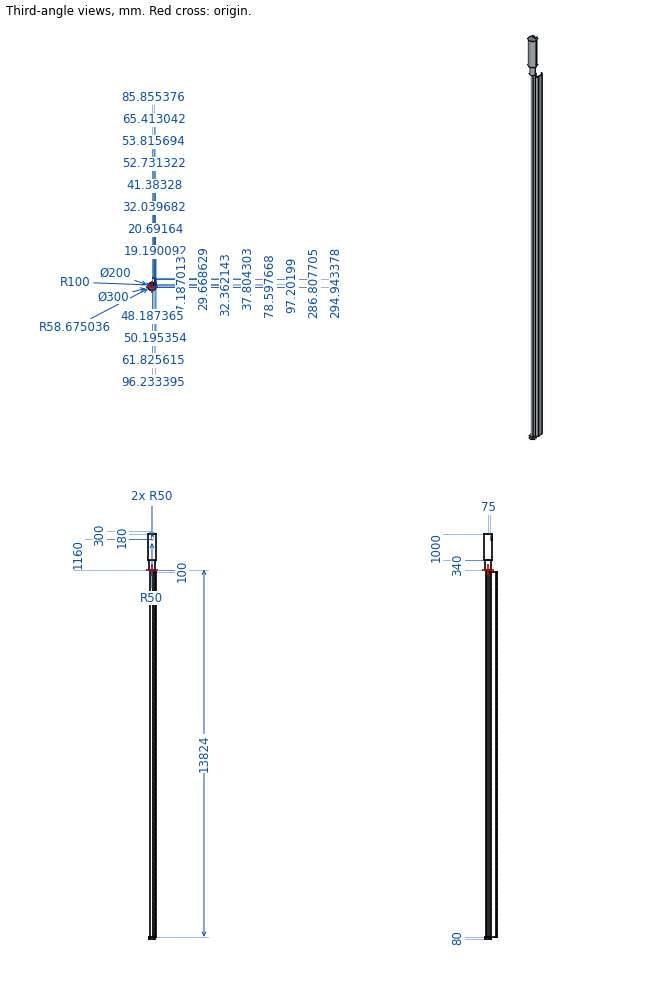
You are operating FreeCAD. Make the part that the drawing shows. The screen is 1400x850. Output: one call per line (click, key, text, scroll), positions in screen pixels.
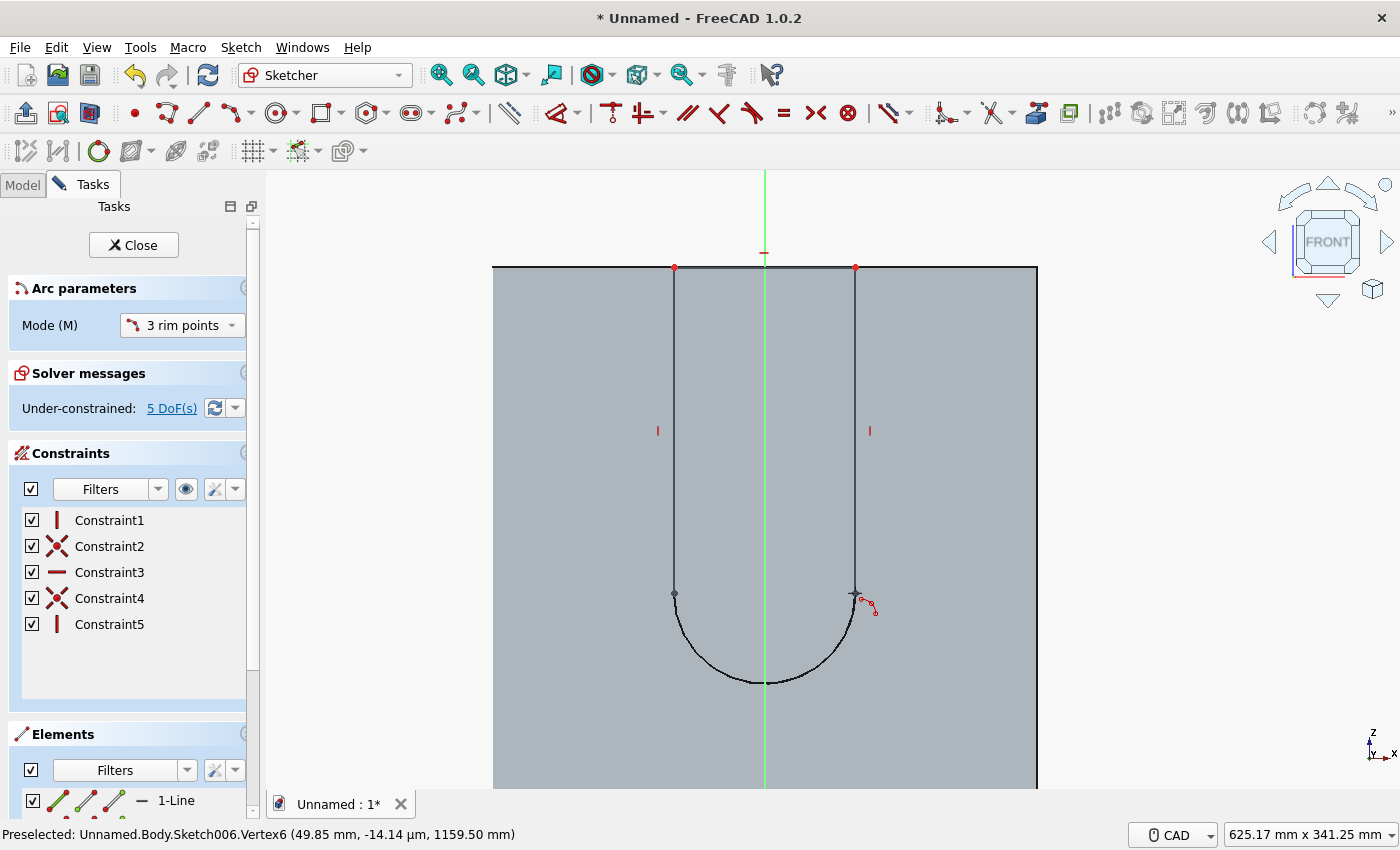
click(855, 594)
click(674, 594)
click(737, 679)
key(Escape)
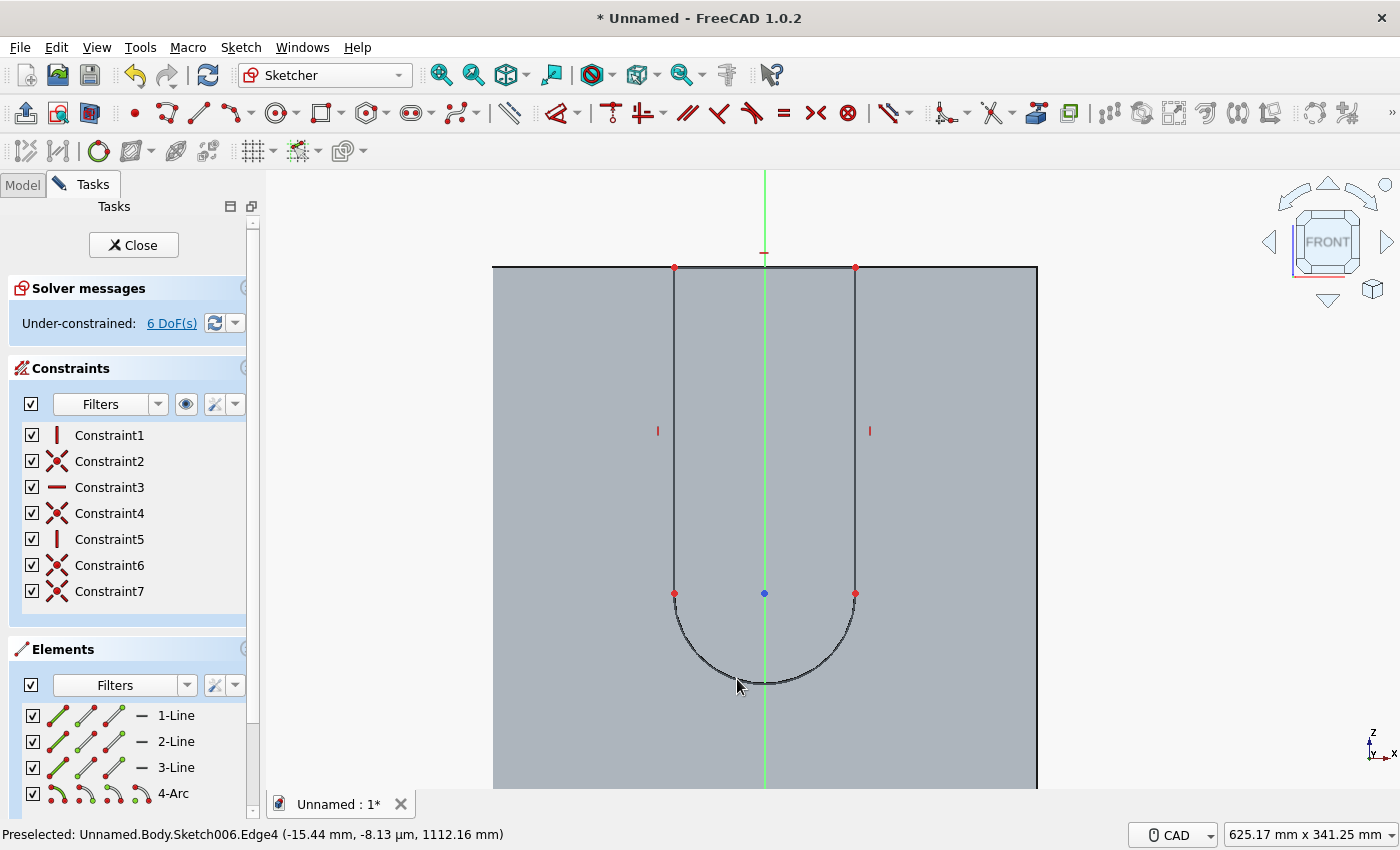
click(764, 594)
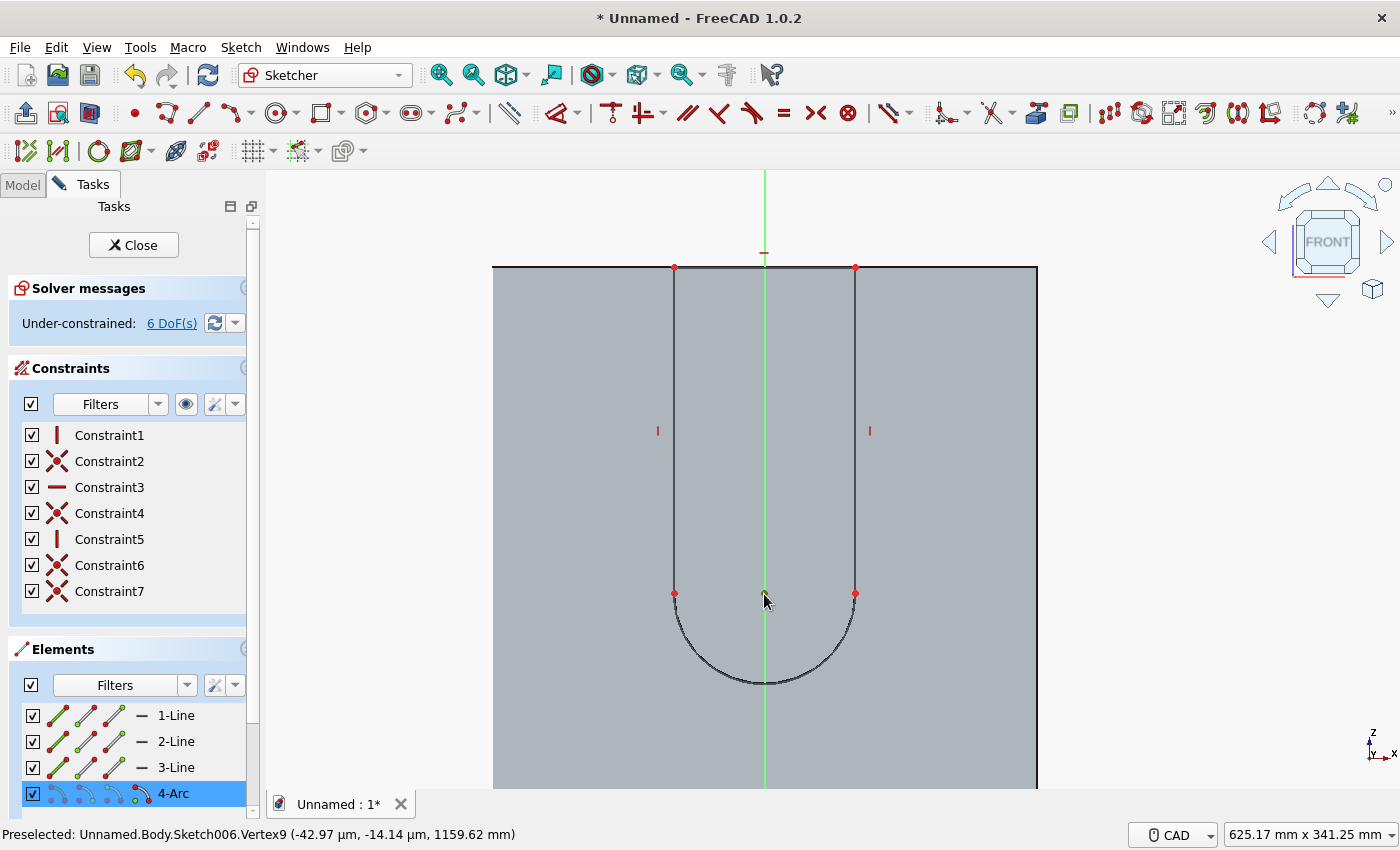
click(765, 721)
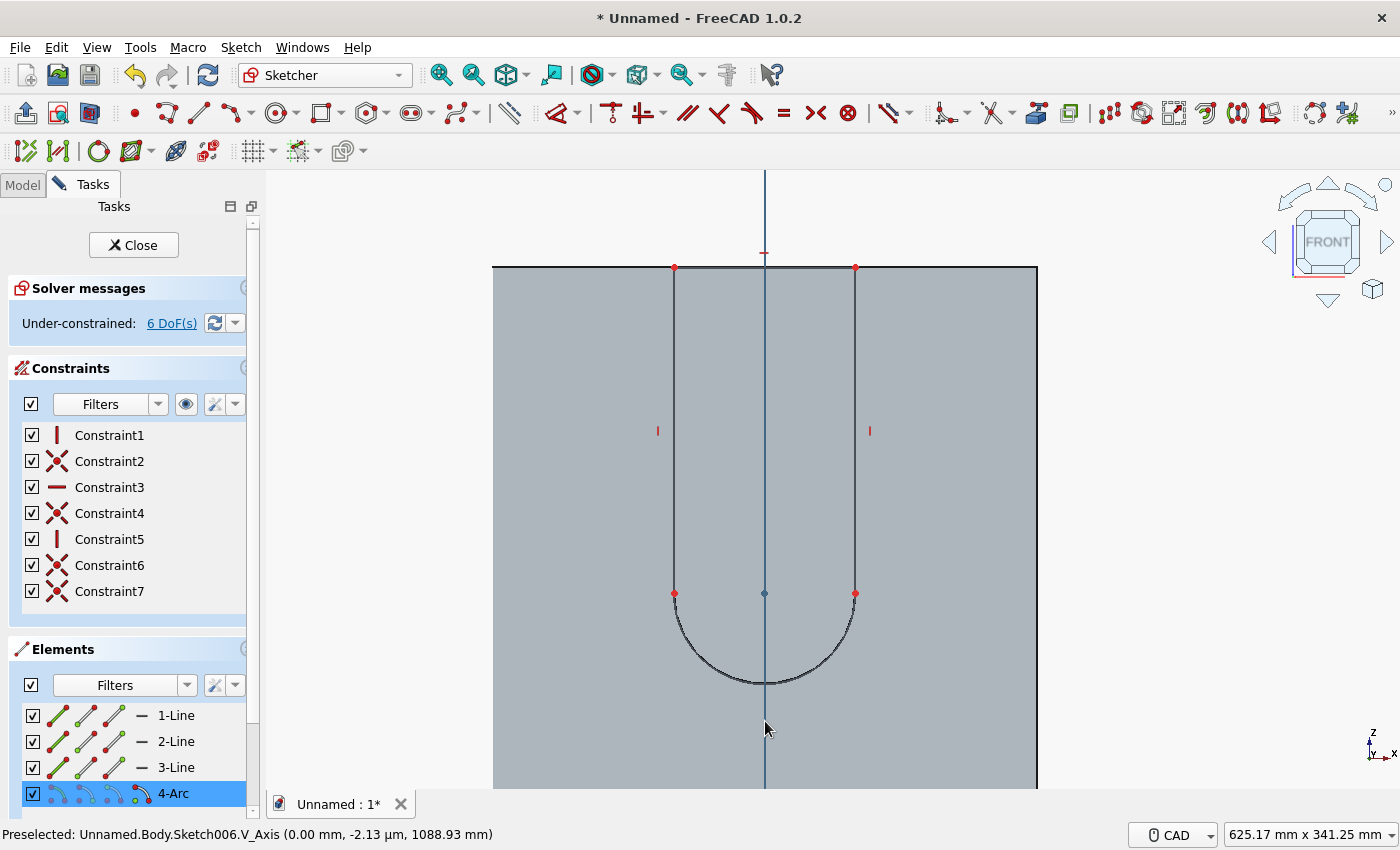
key(c)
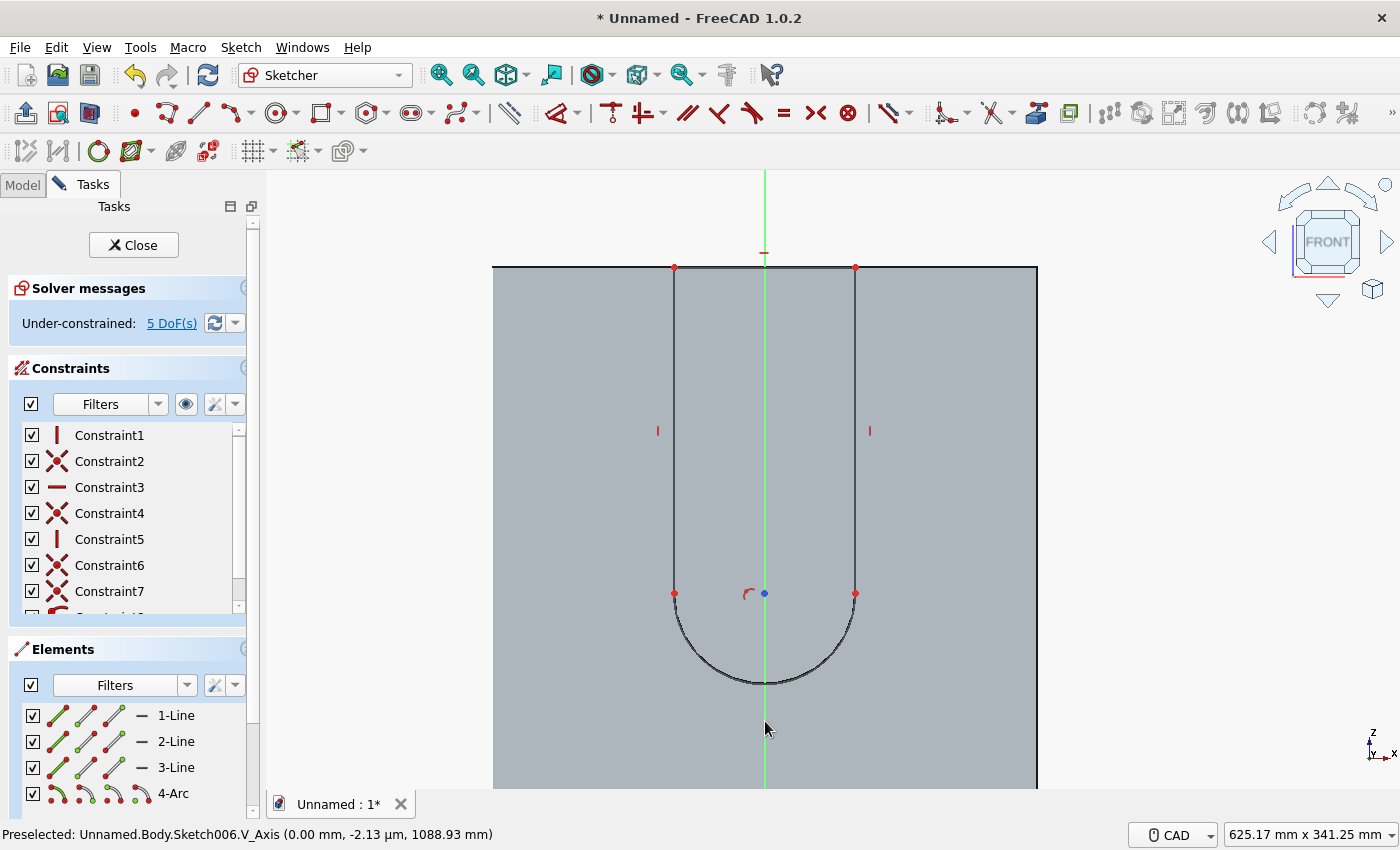
key(d)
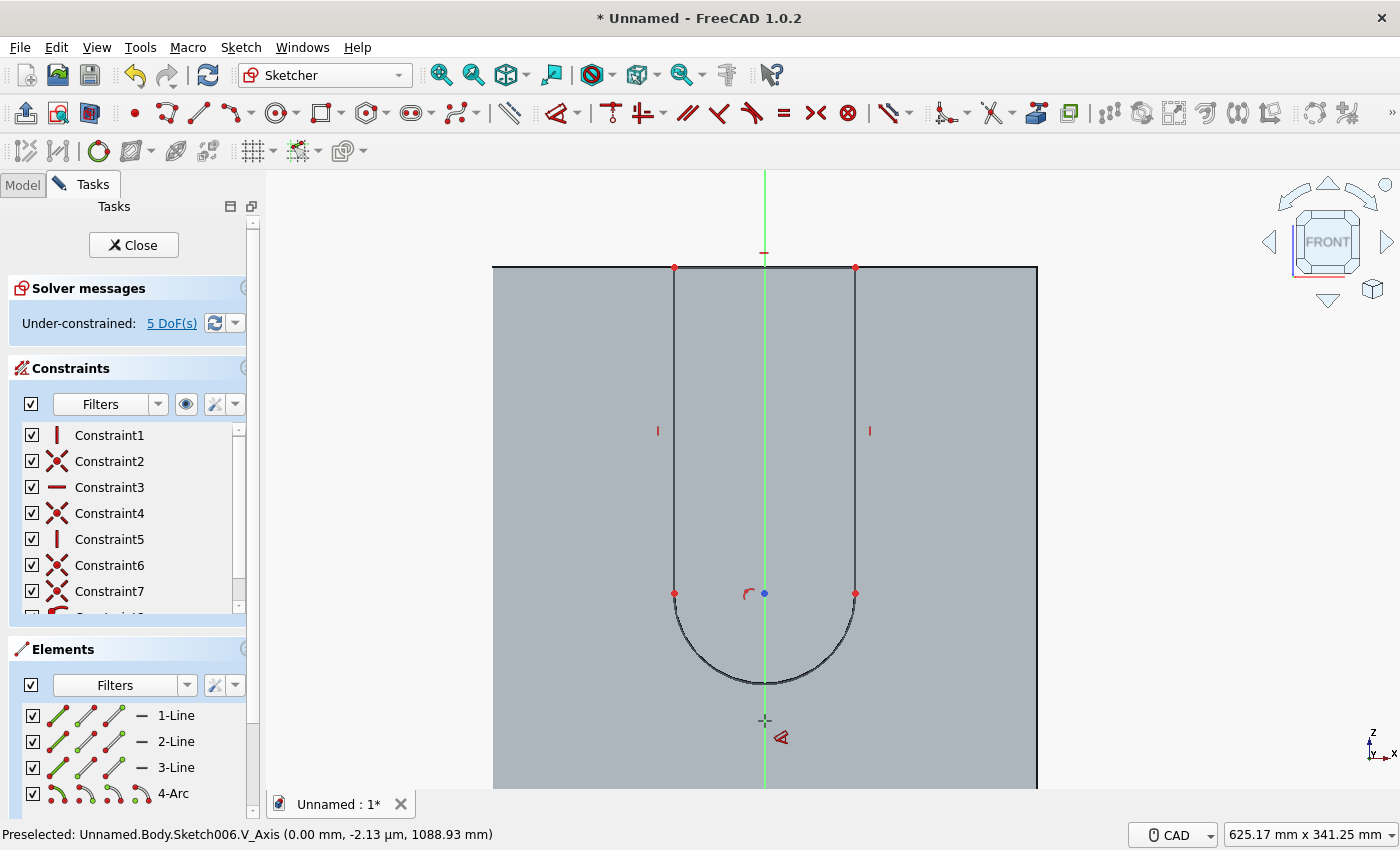
click(711, 667)
click(692, 693)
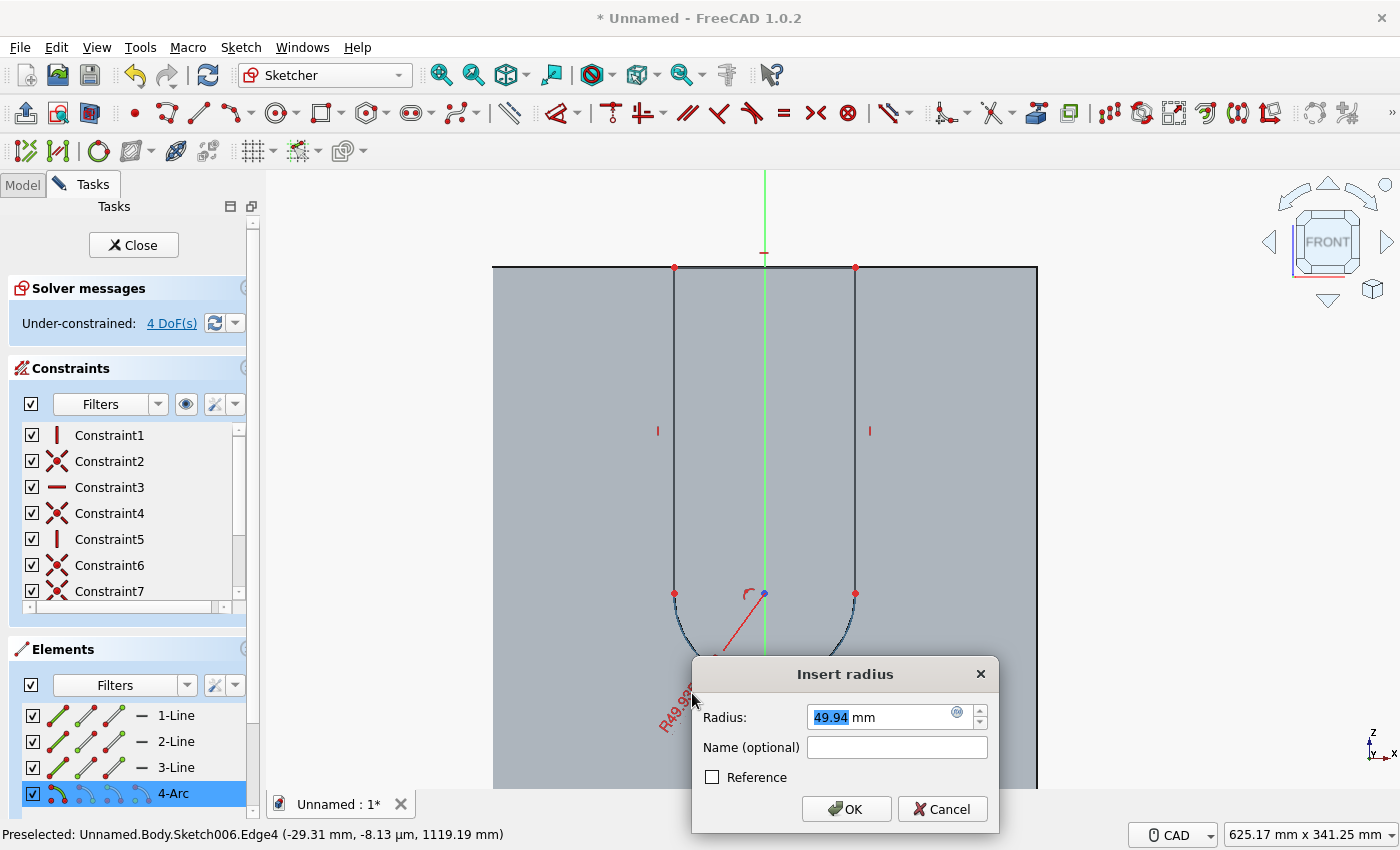
text(50)
key(Return)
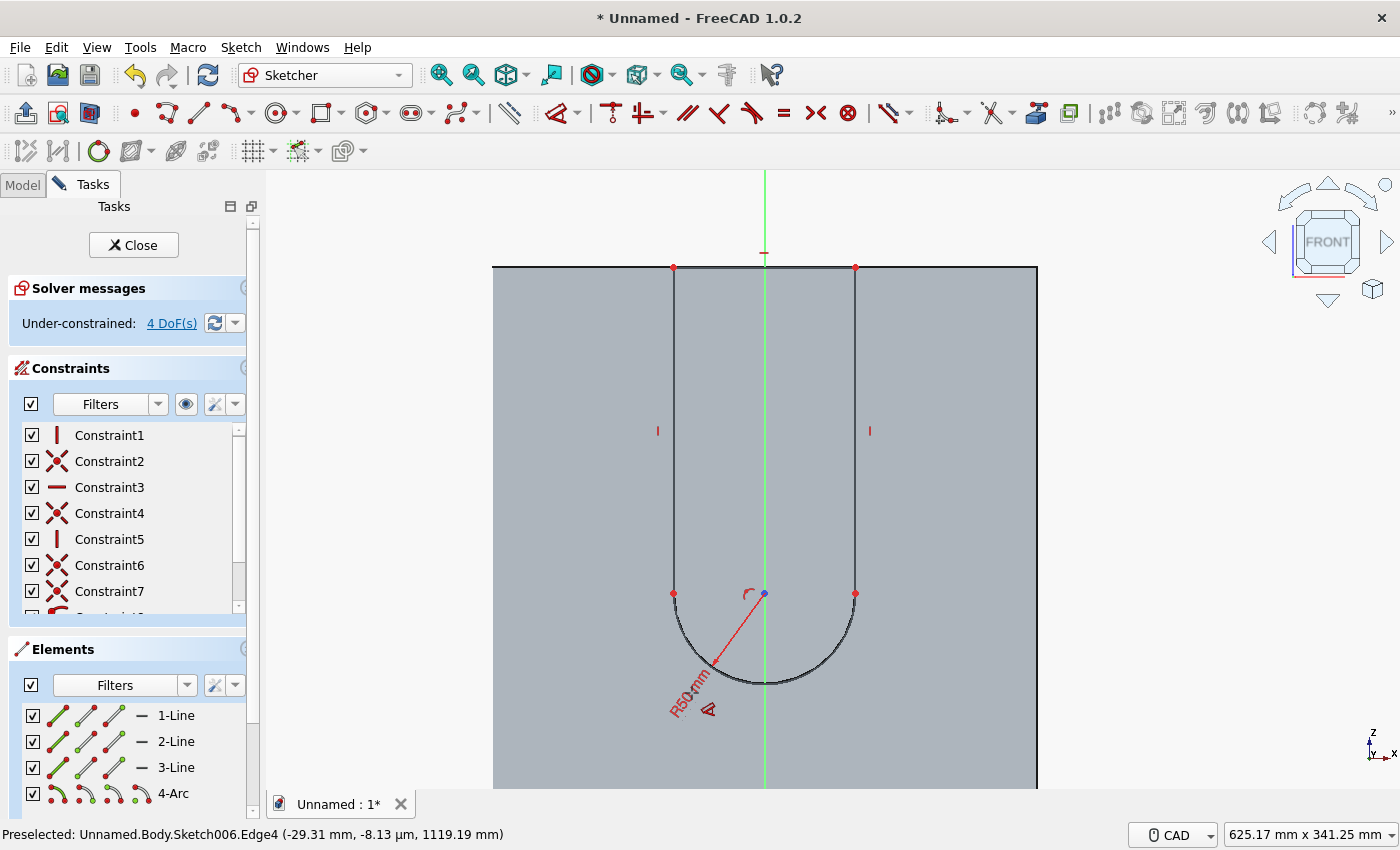
click(674, 496)
click(640, 431)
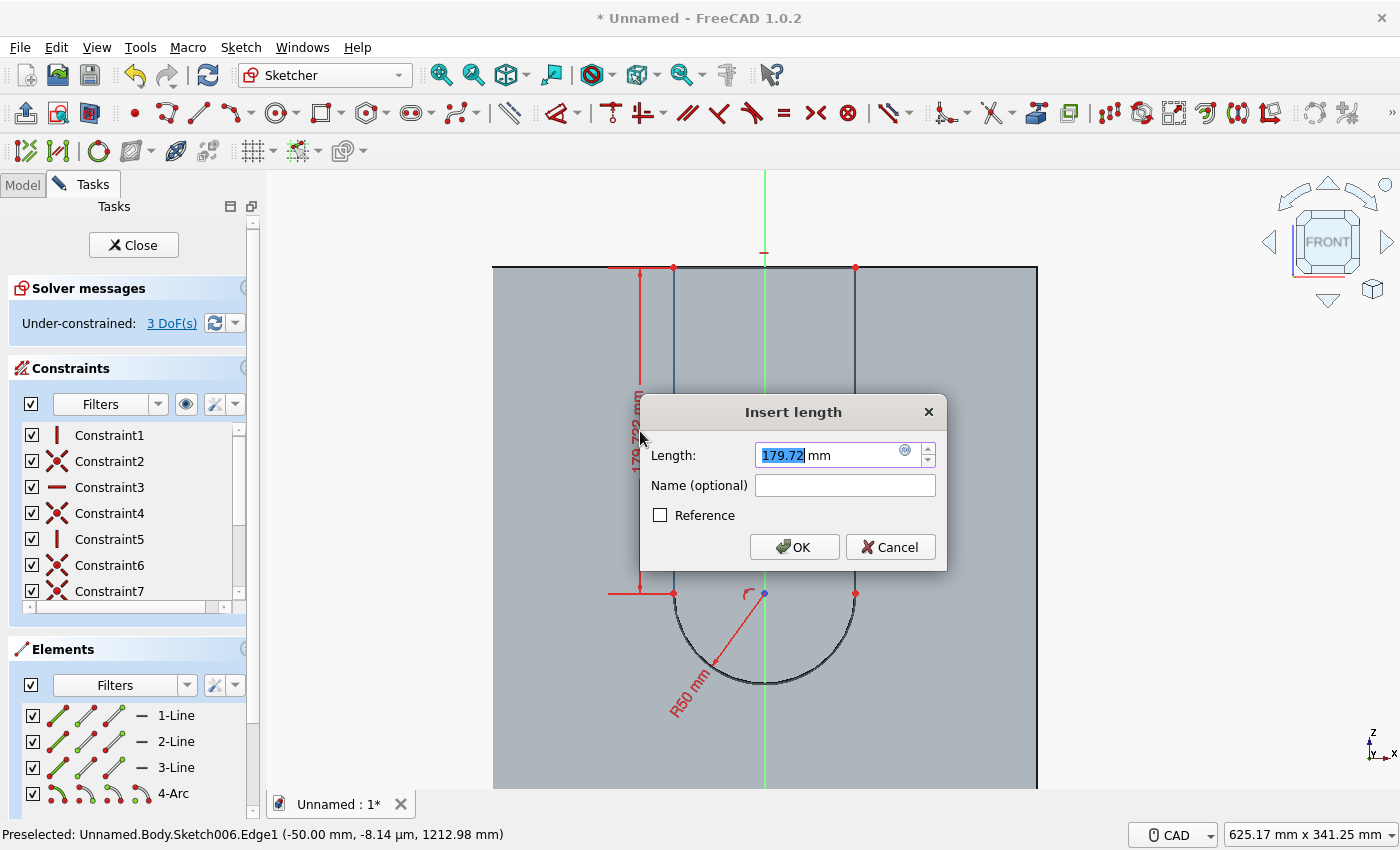
text(180)
key(Return)